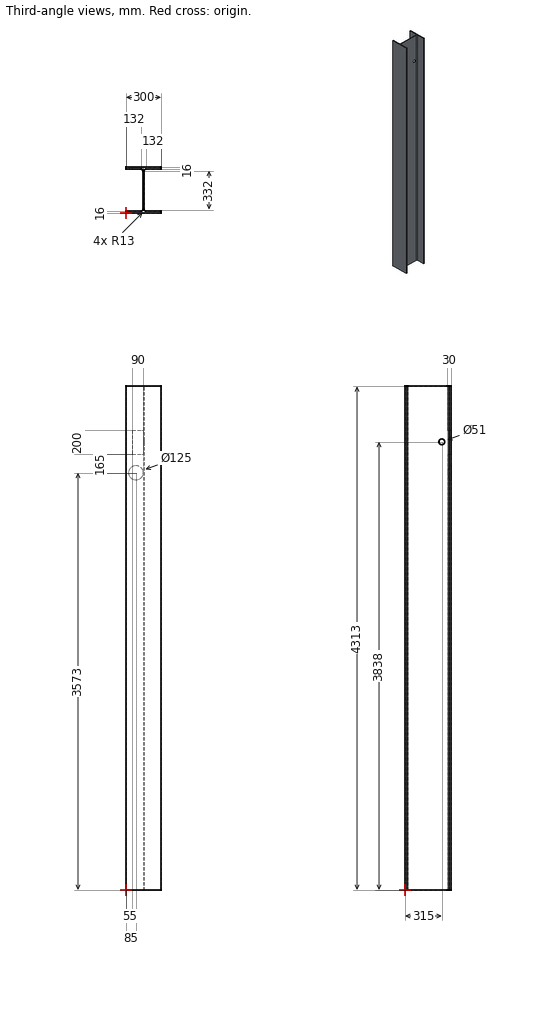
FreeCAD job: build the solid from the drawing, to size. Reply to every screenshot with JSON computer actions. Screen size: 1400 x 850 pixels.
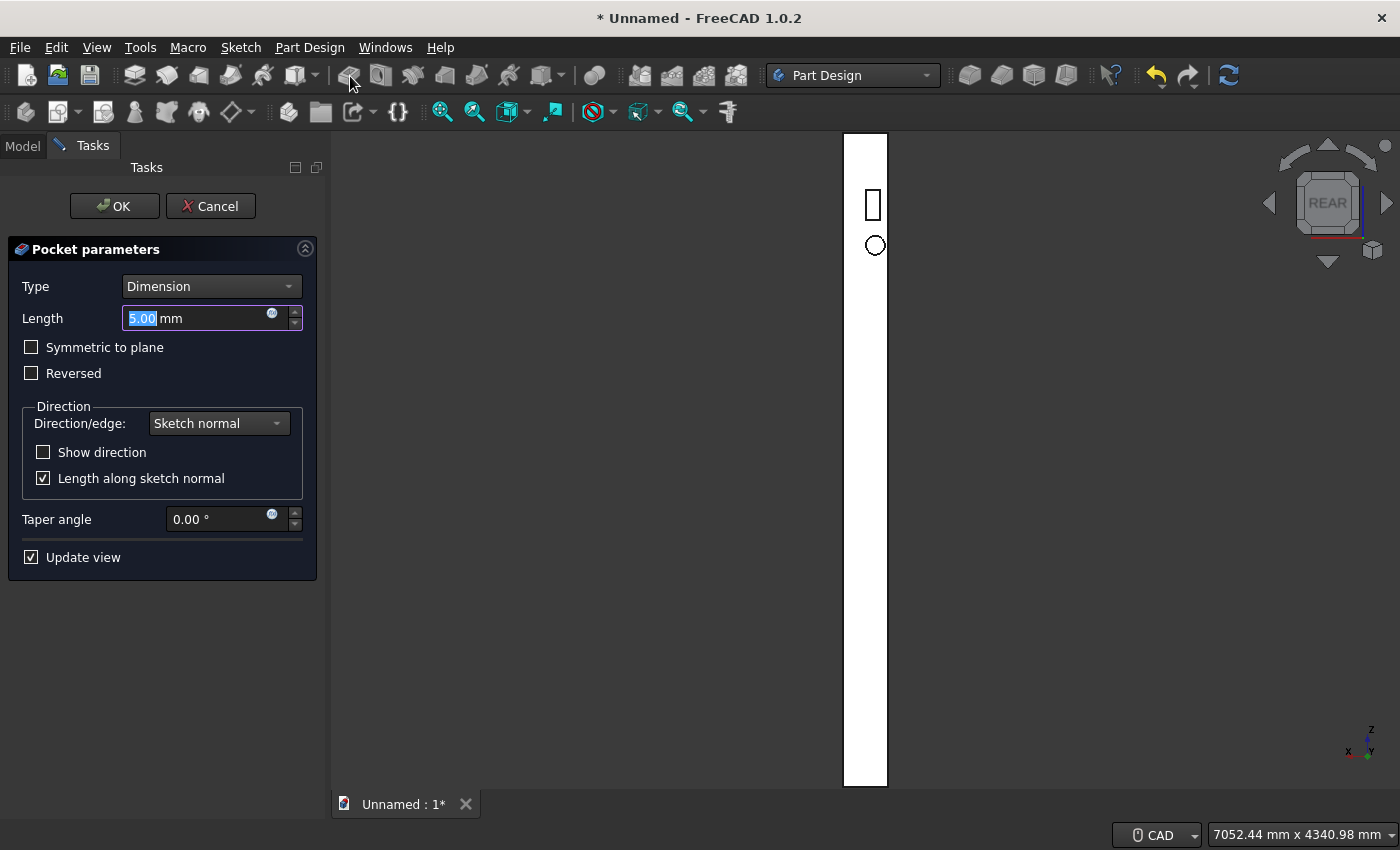
{"action": "type", "text": "30"}
{"action": "key", "text": "Tab"}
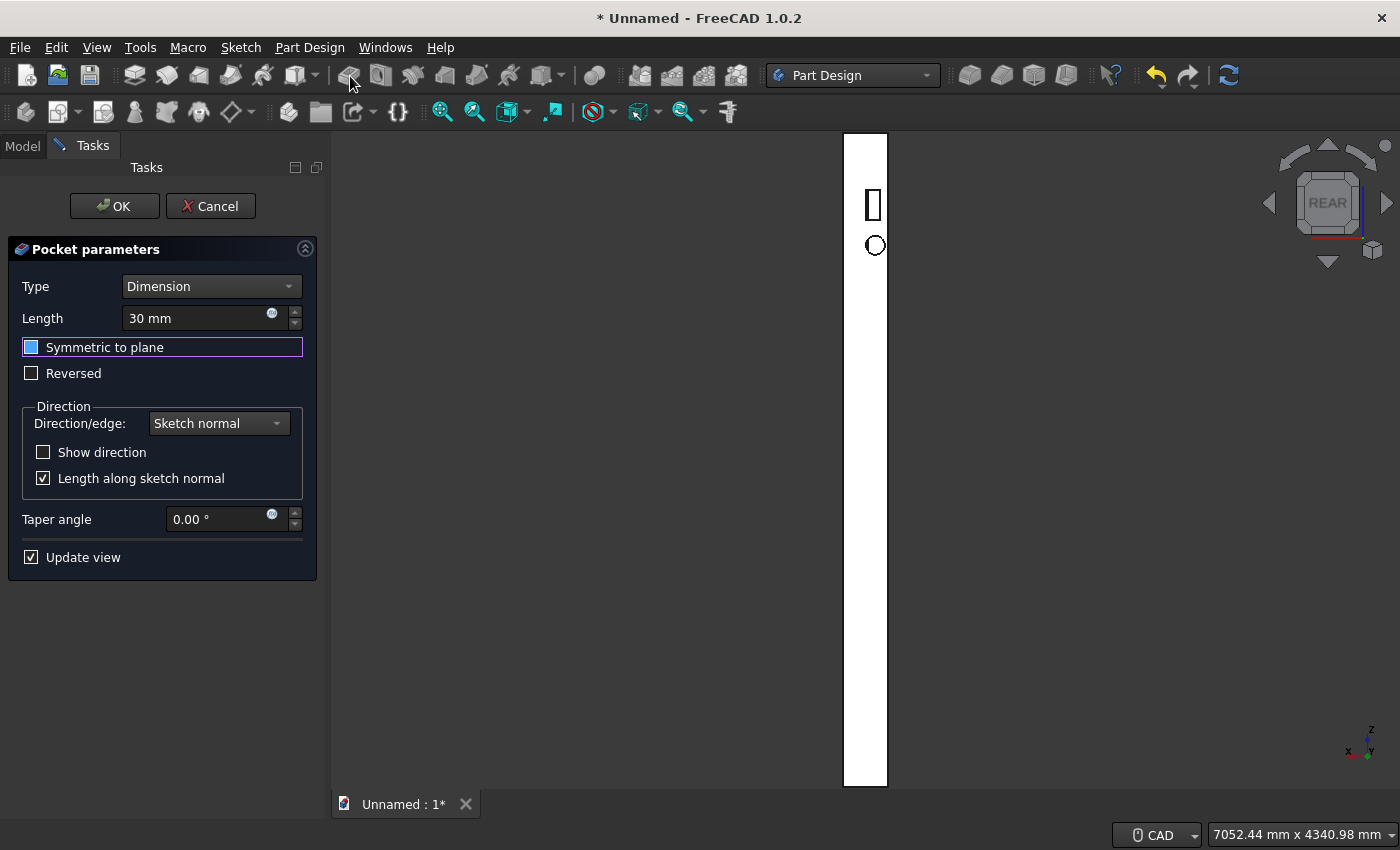
{"action": "left_click", "coordinate": [115, 206]}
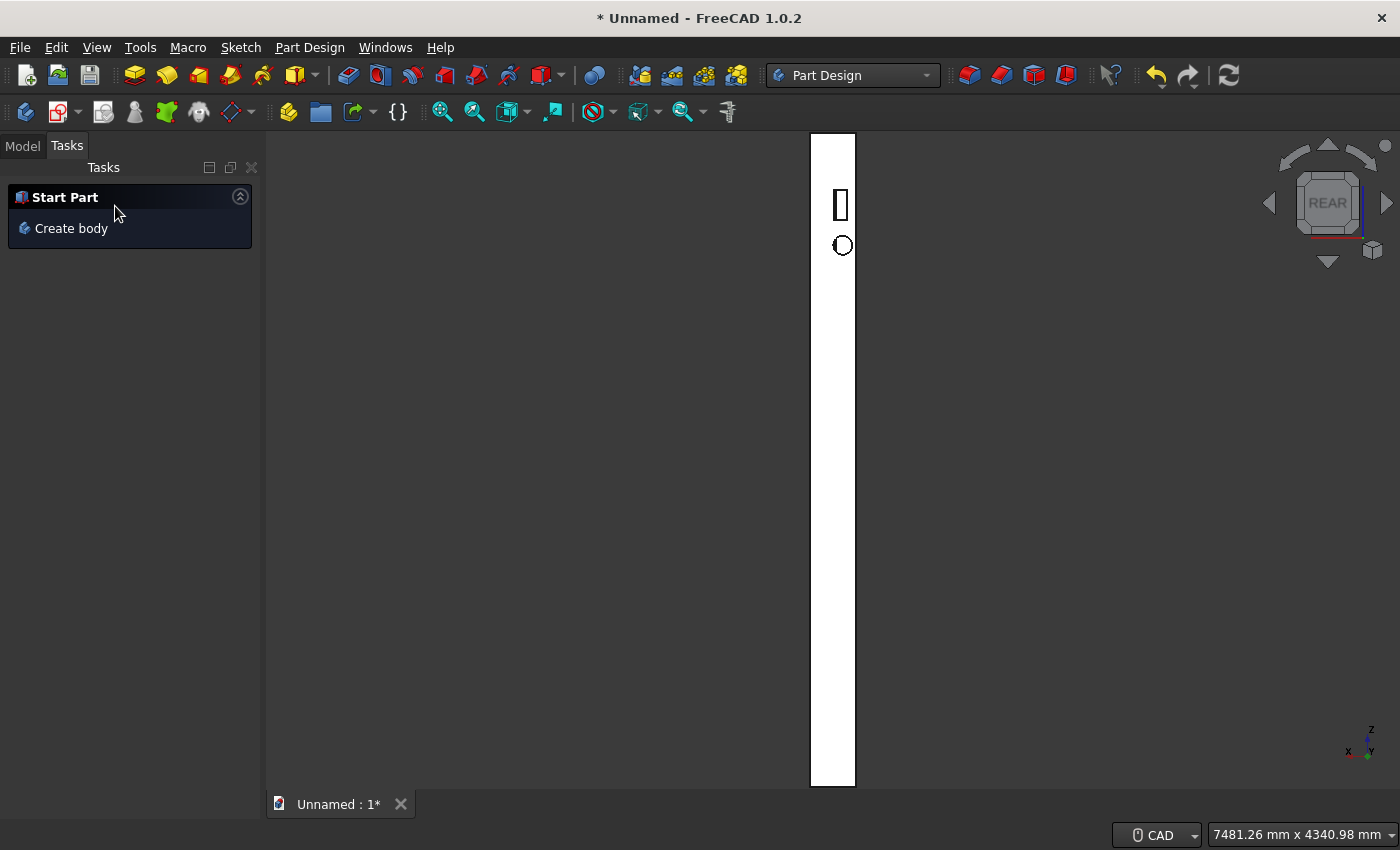
{"action": "key", "text": "6"}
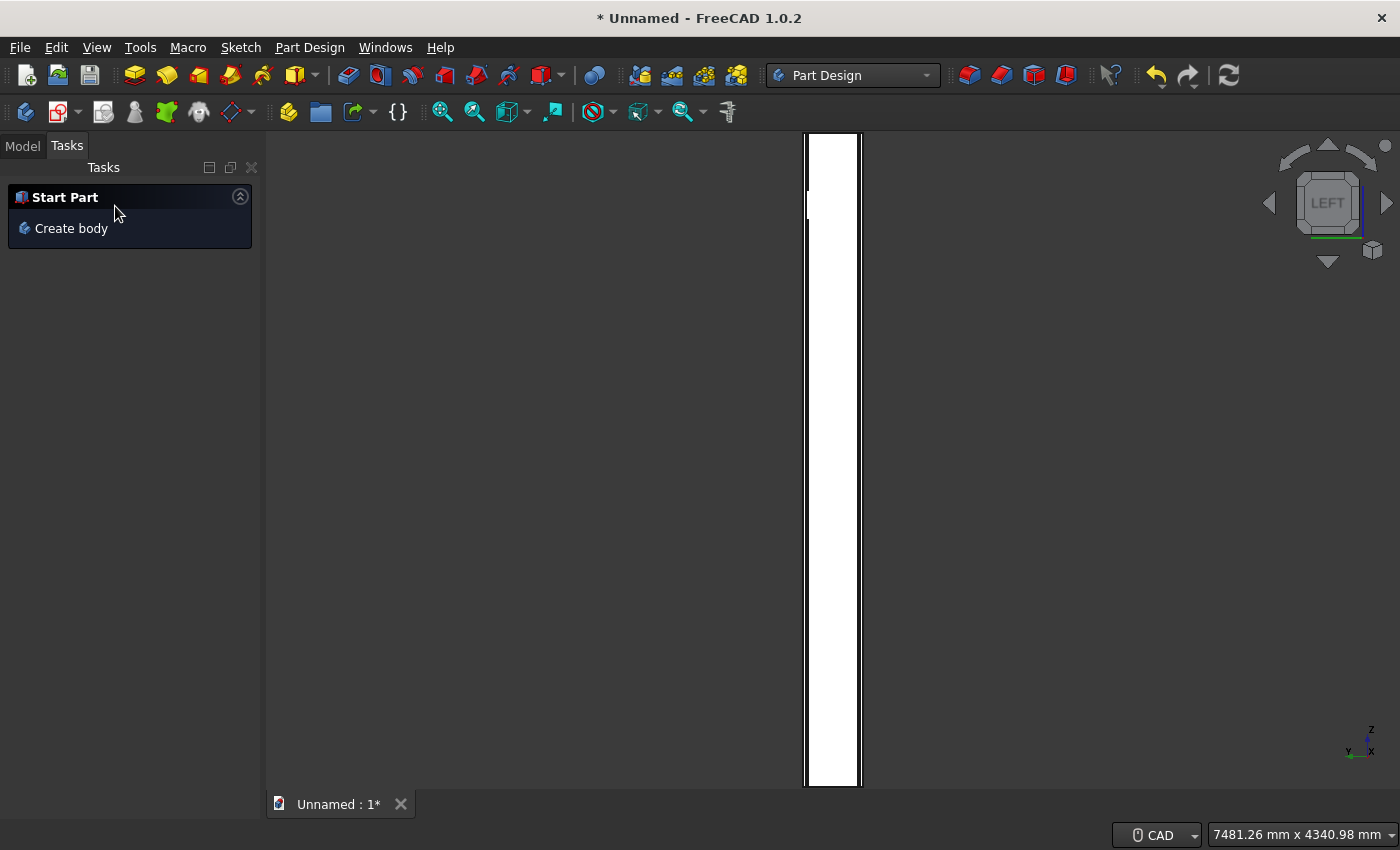
{"action": "left_click", "coordinate": [831, 179]}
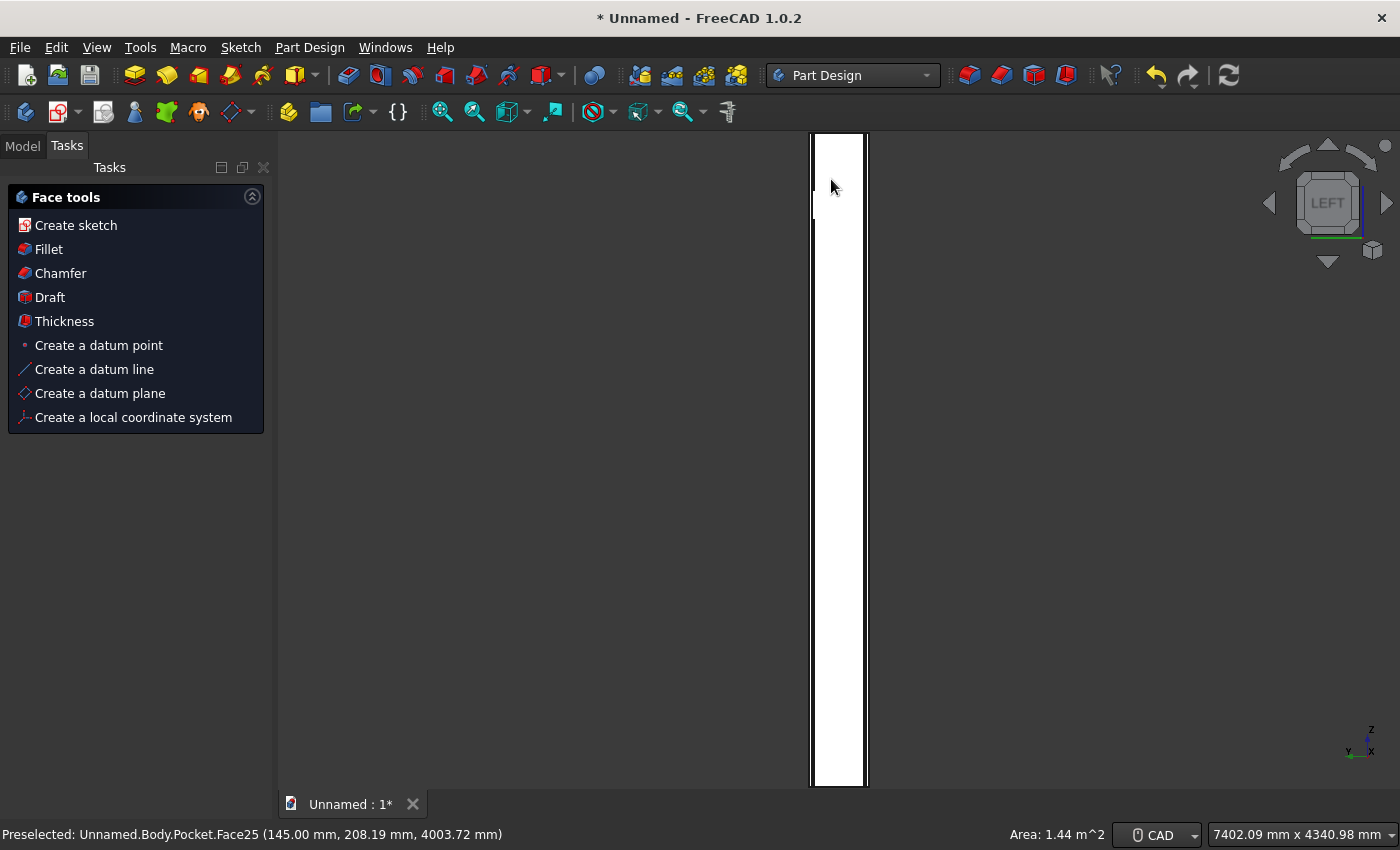
{"action": "left_click", "coordinate": [58, 112]}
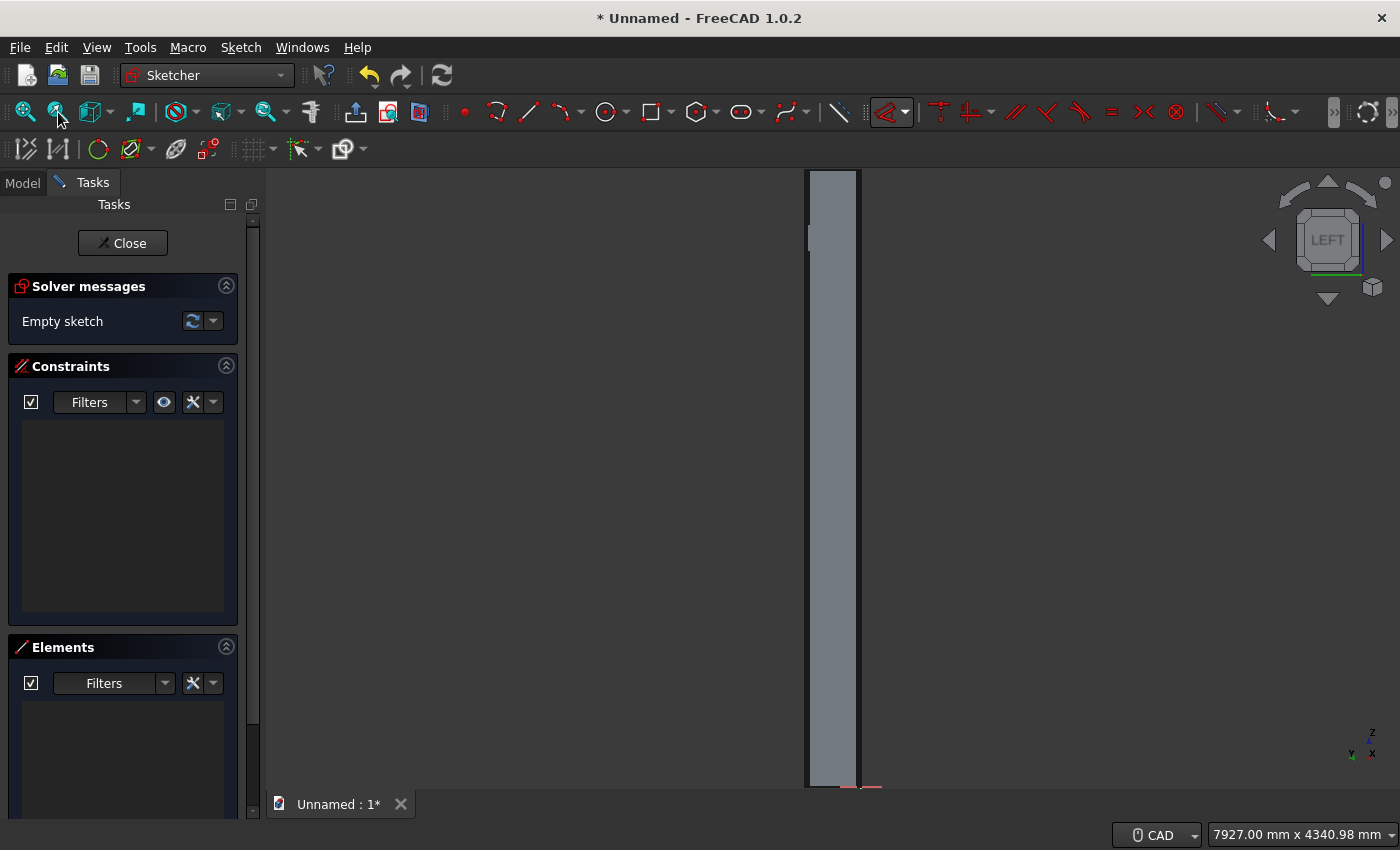
{"action": "left_click", "coordinate": [420, 112]}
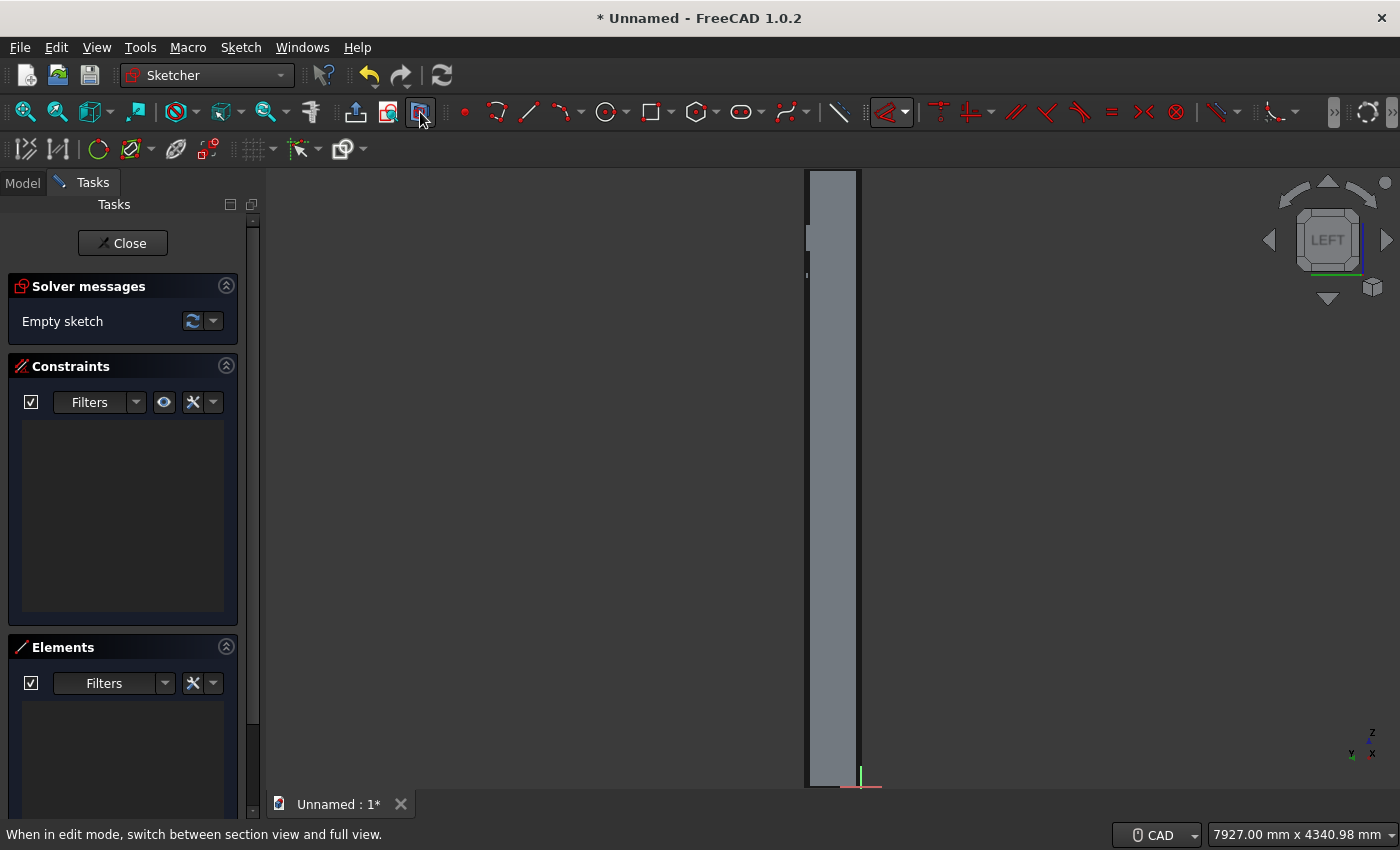
{"action": "scroll", "coordinate": [819, 225], "scroll_direction": "up", "scroll_amount": 15}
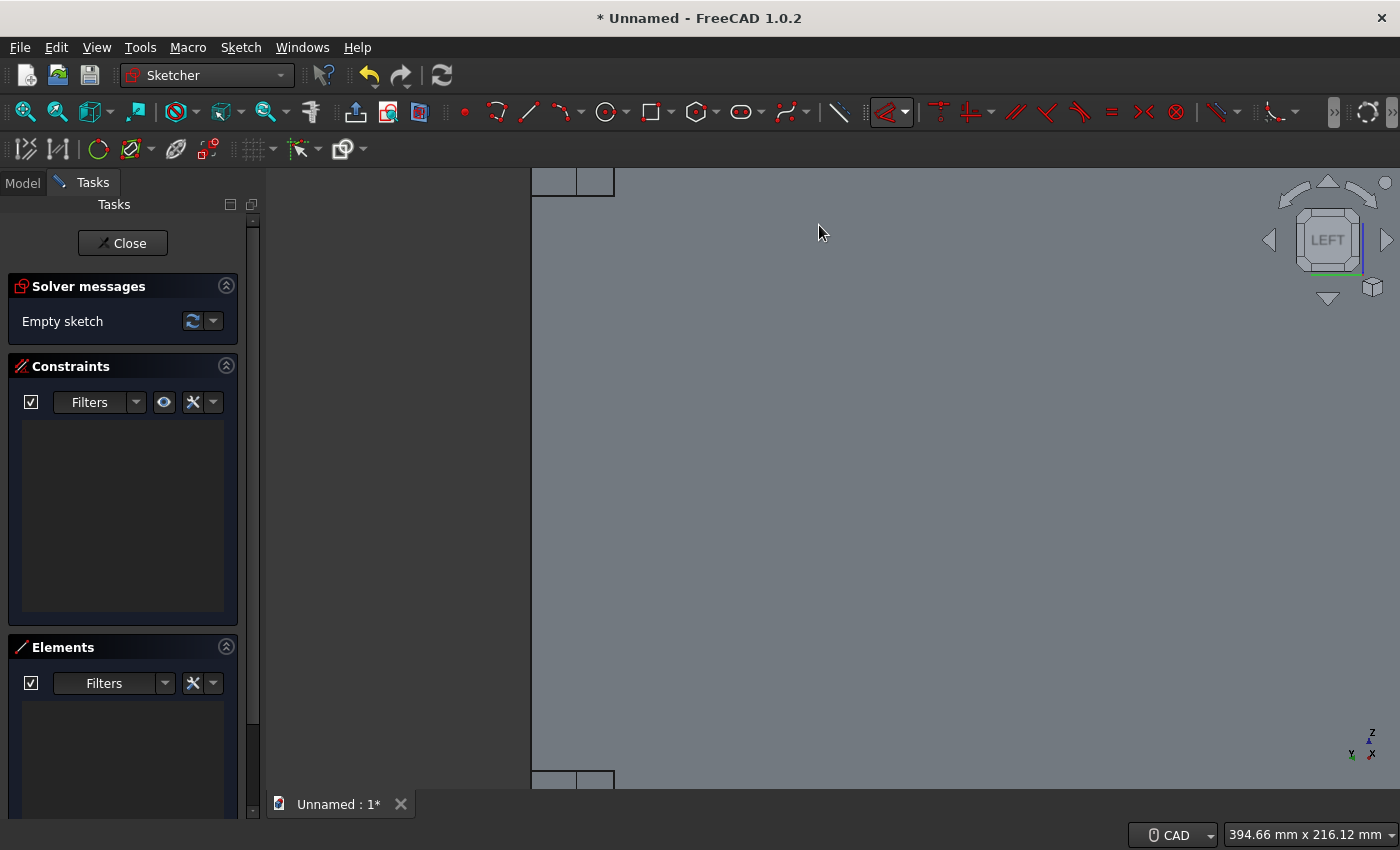
{"action": "scroll", "coordinate": [735, 486], "scroll_direction": "up", "scroll_amount": 5}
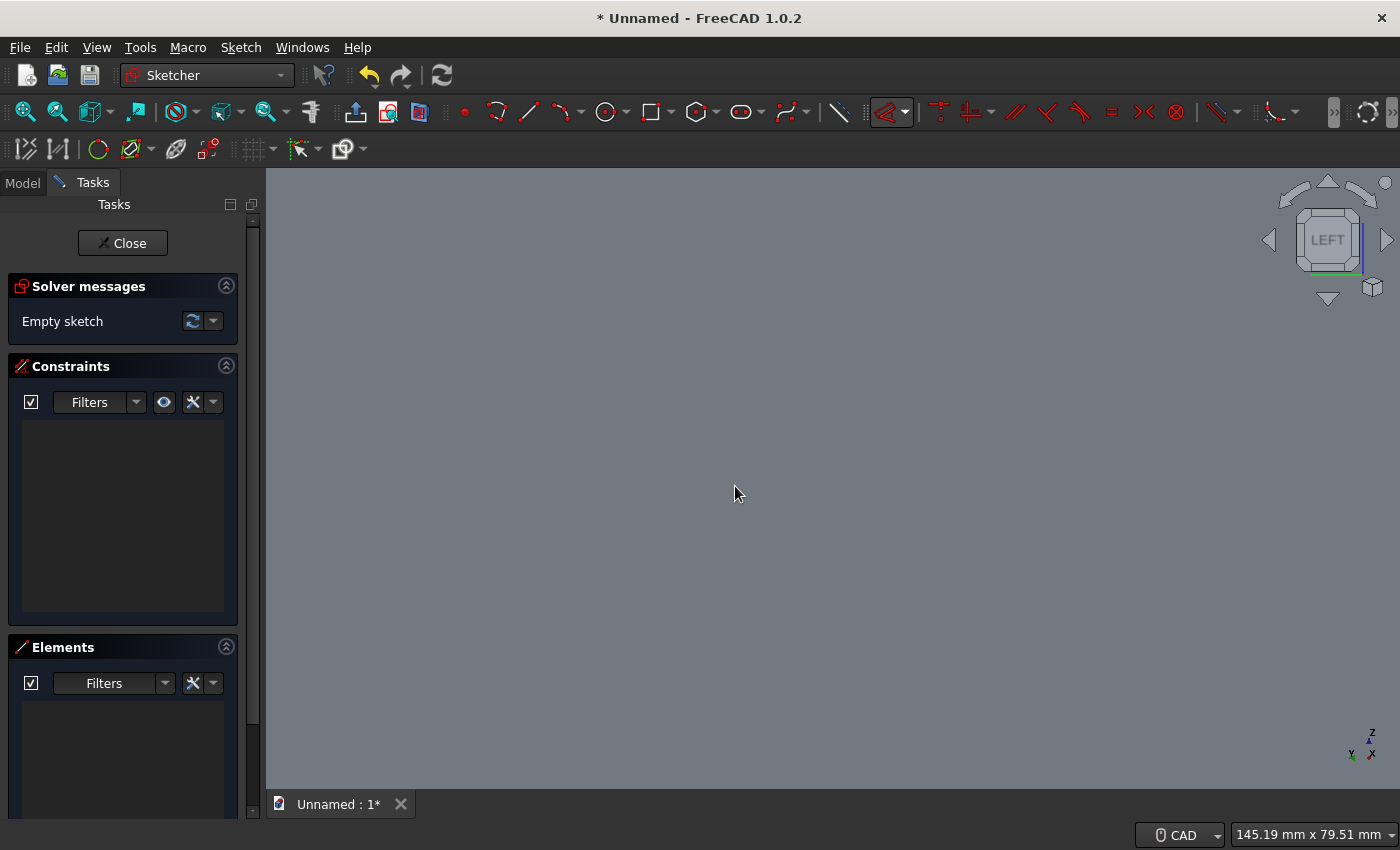
{"action": "left_click", "coordinate": [606, 112]}